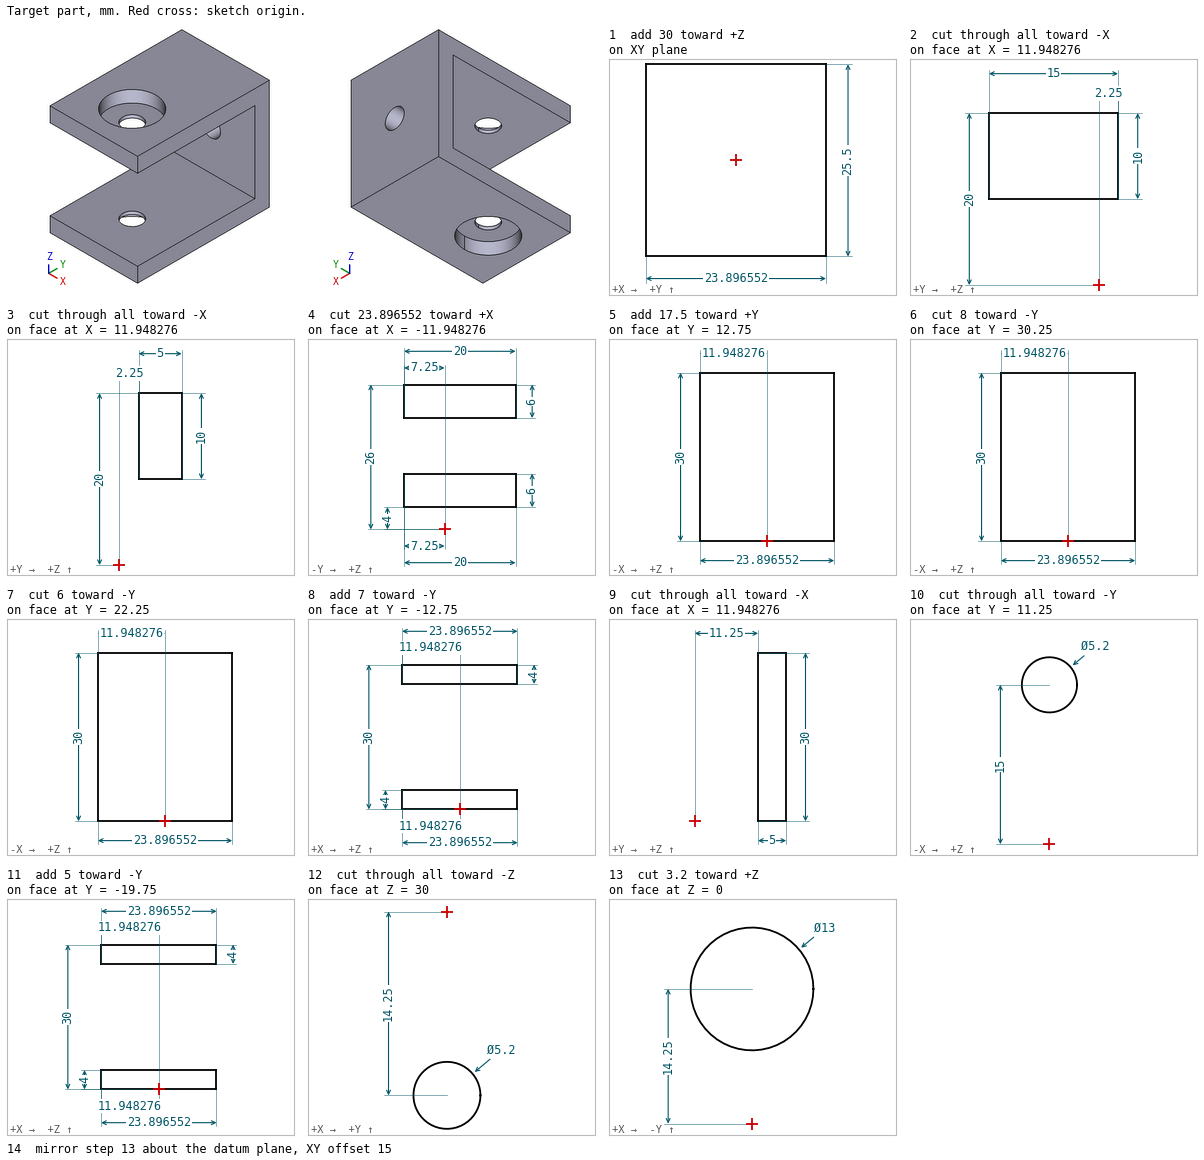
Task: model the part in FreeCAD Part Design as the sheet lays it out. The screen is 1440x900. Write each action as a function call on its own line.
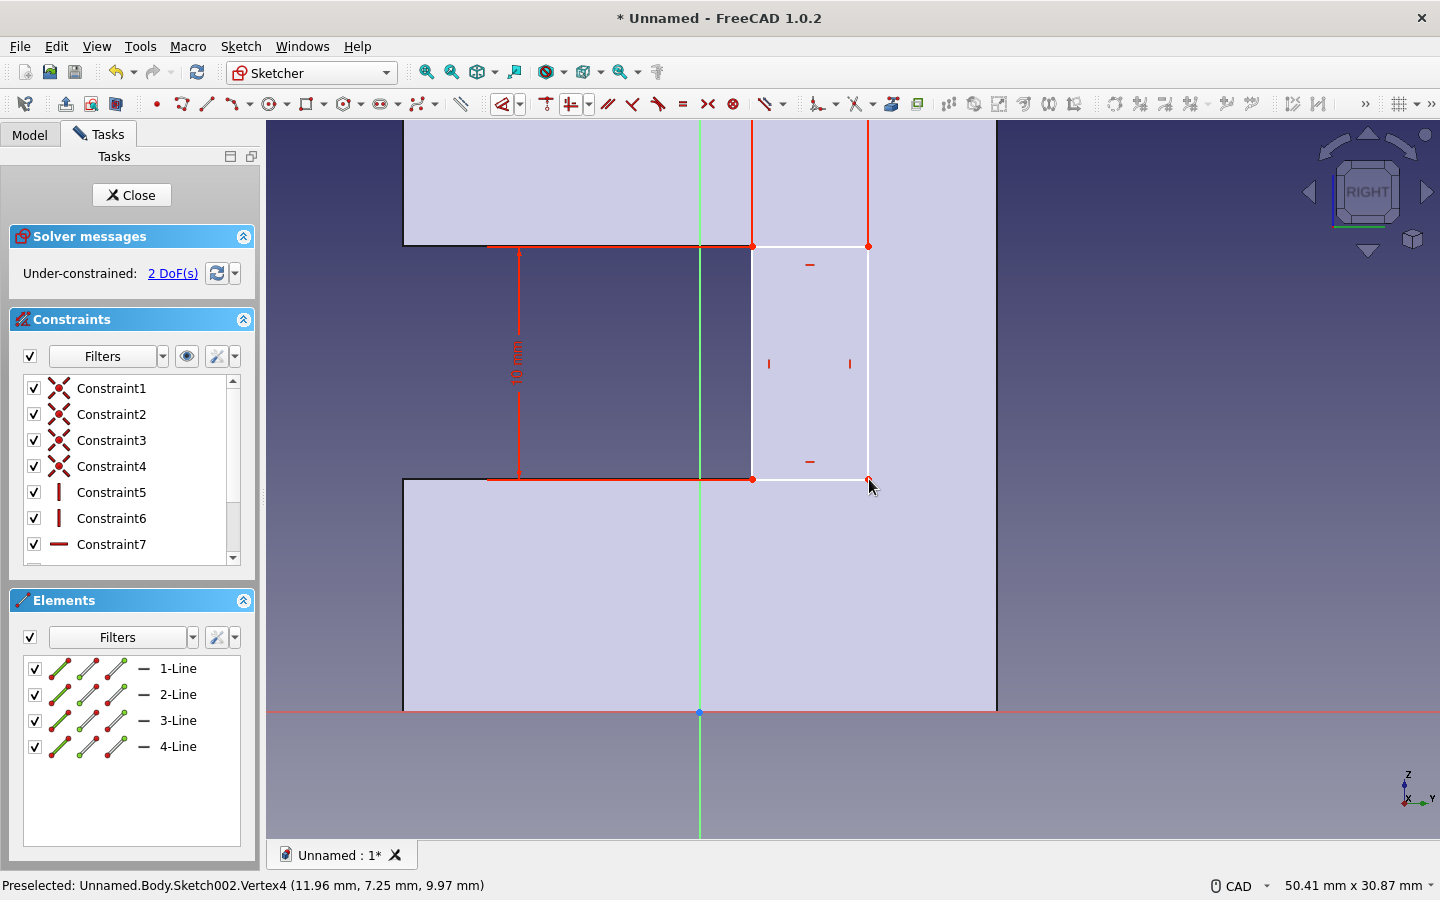
click(502, 104)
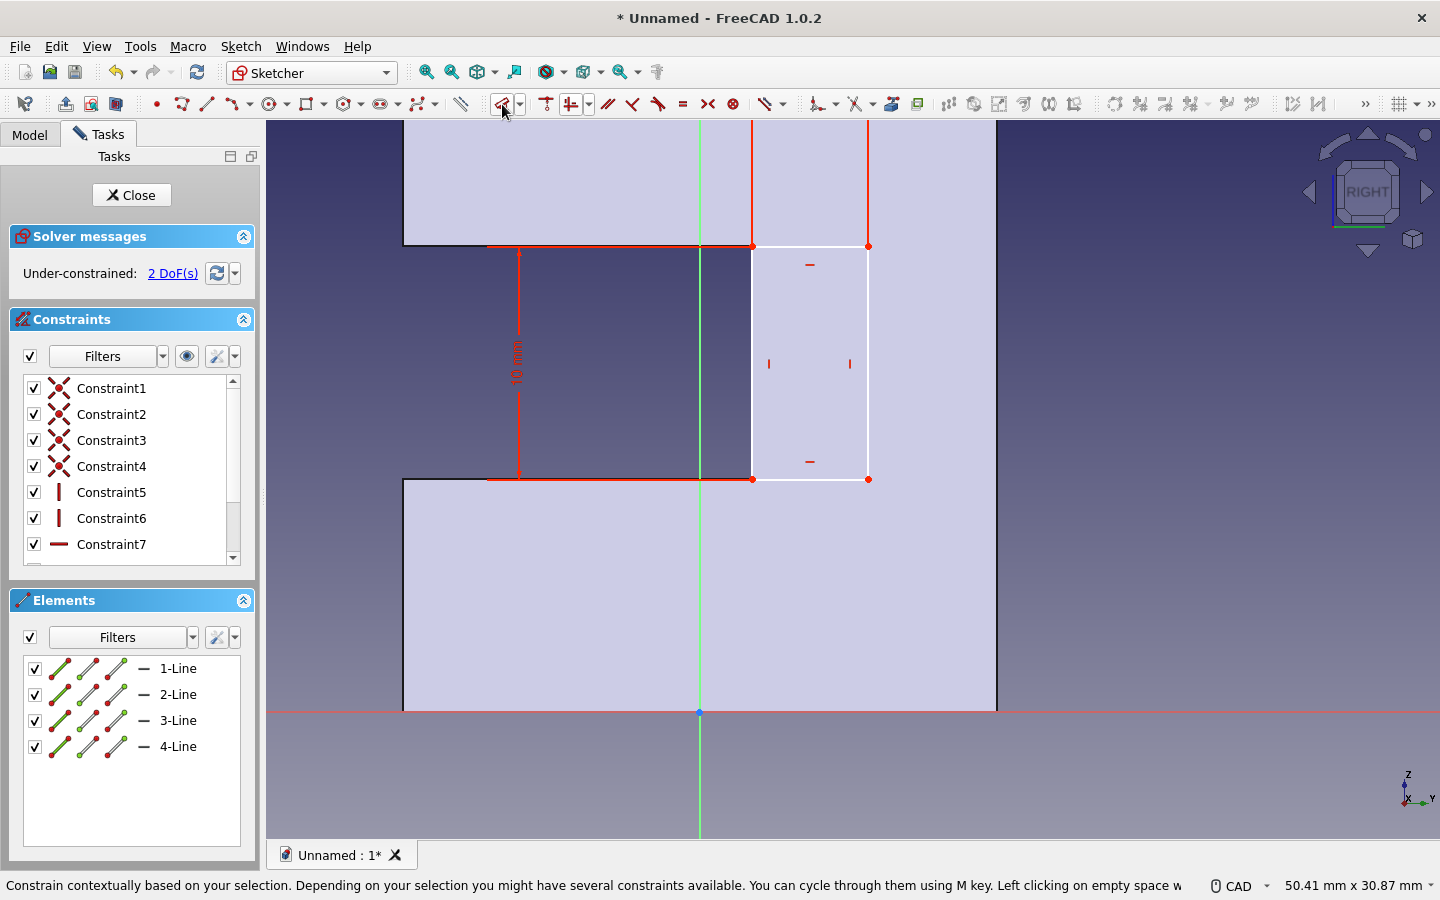
click(752, 247)
click(666, 480)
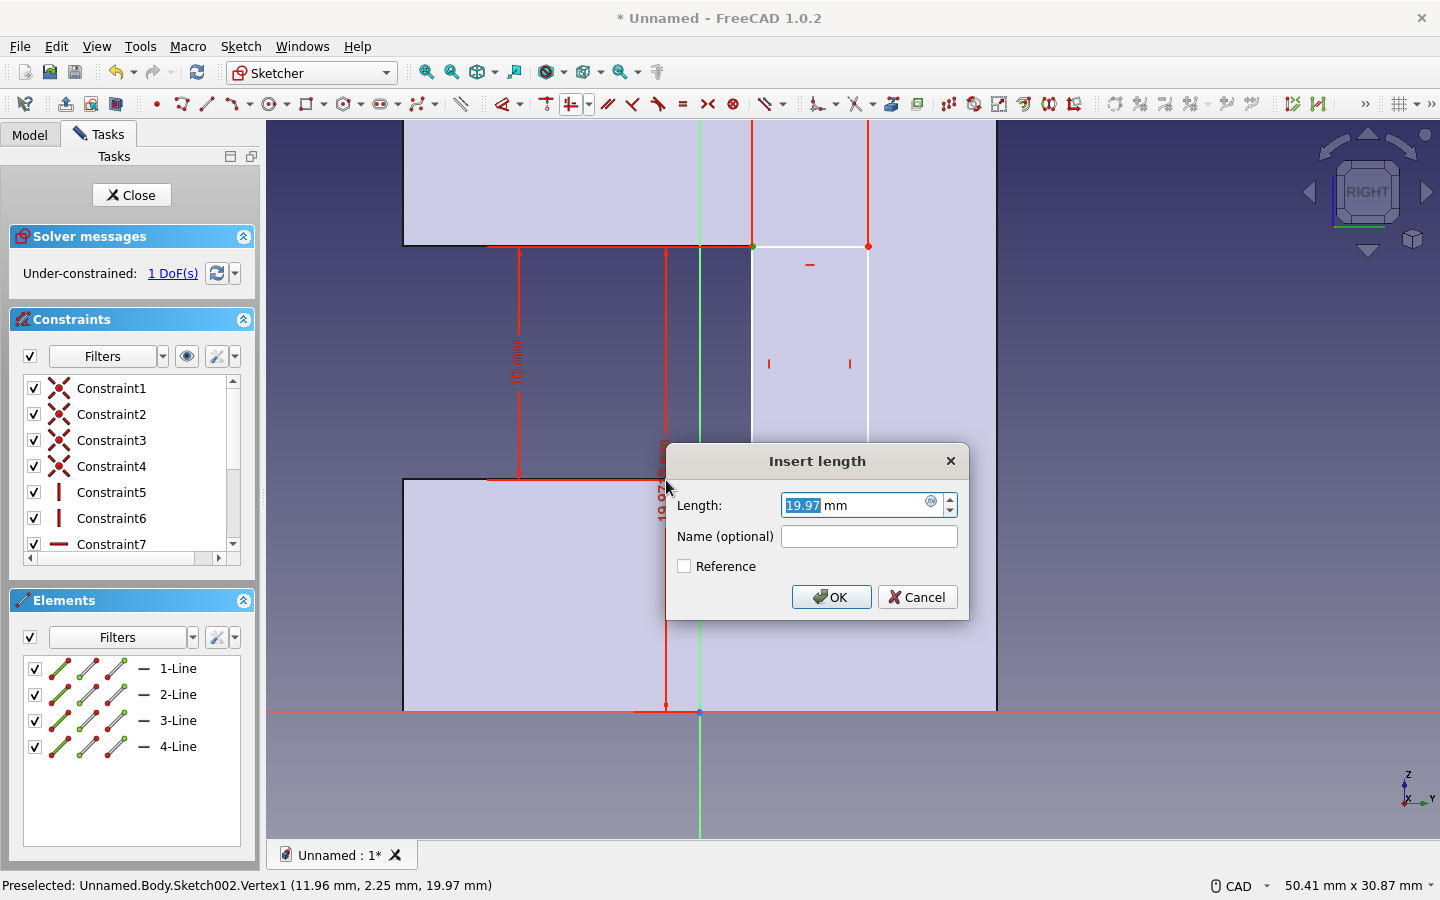
text(20)
key(Return)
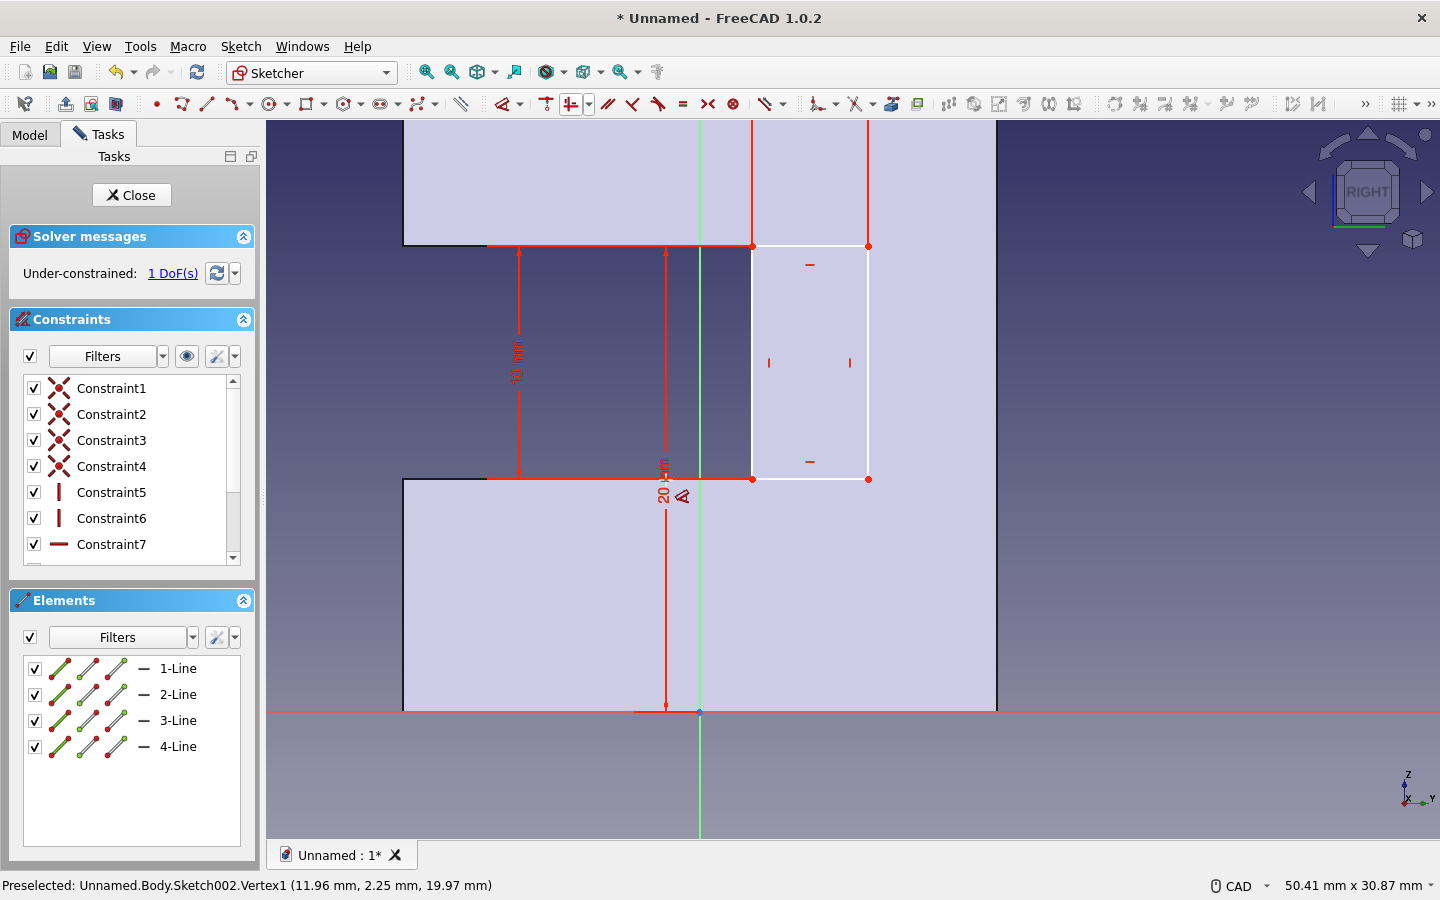
click(752, 246)
click(726, 746)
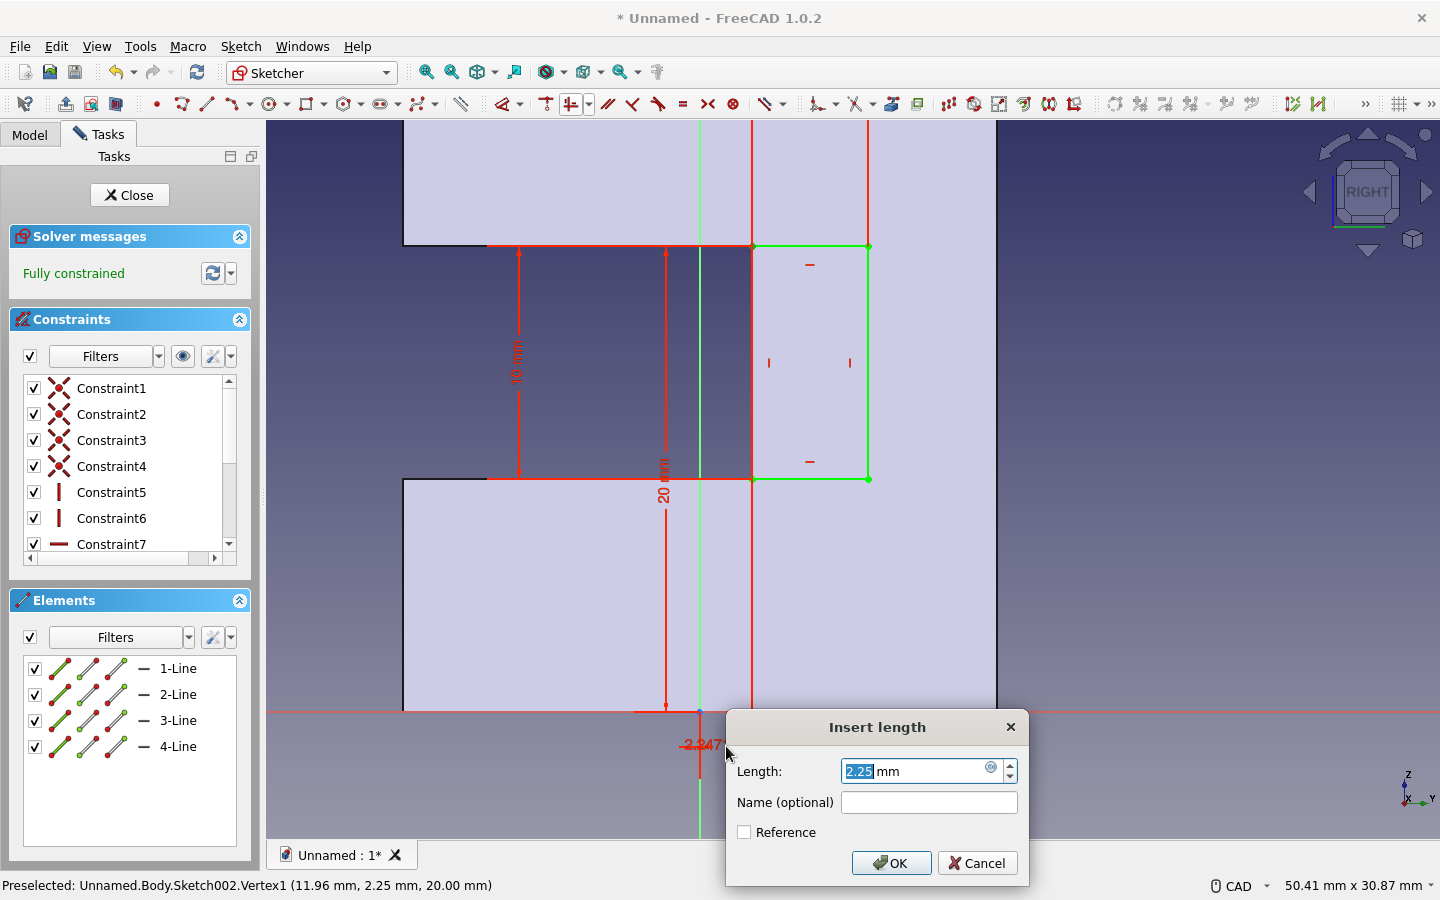
text(2.25)
key(Return)
key(Escape)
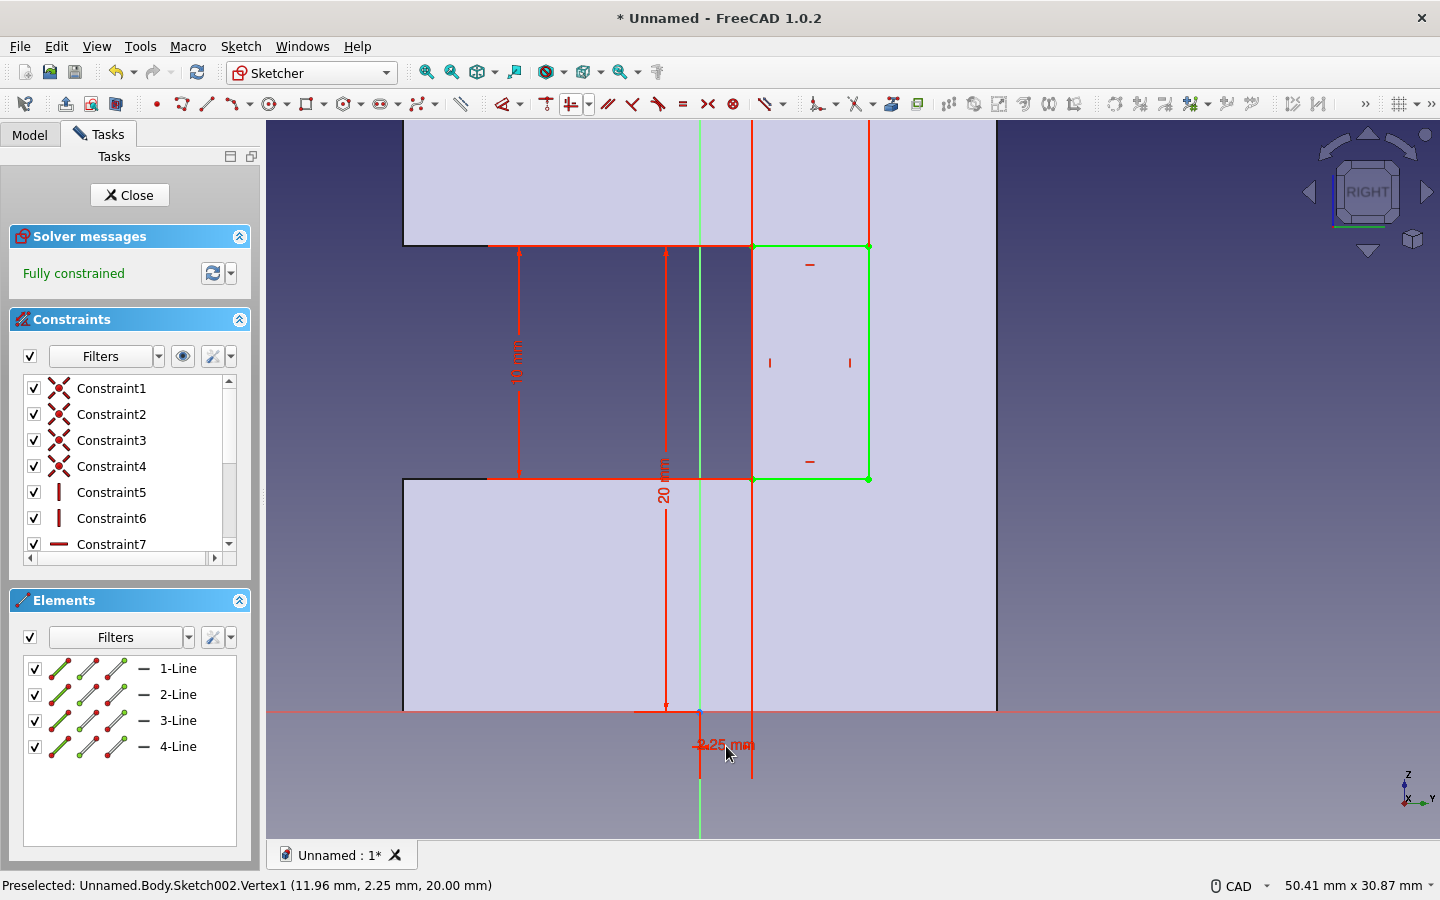
click(130, 195)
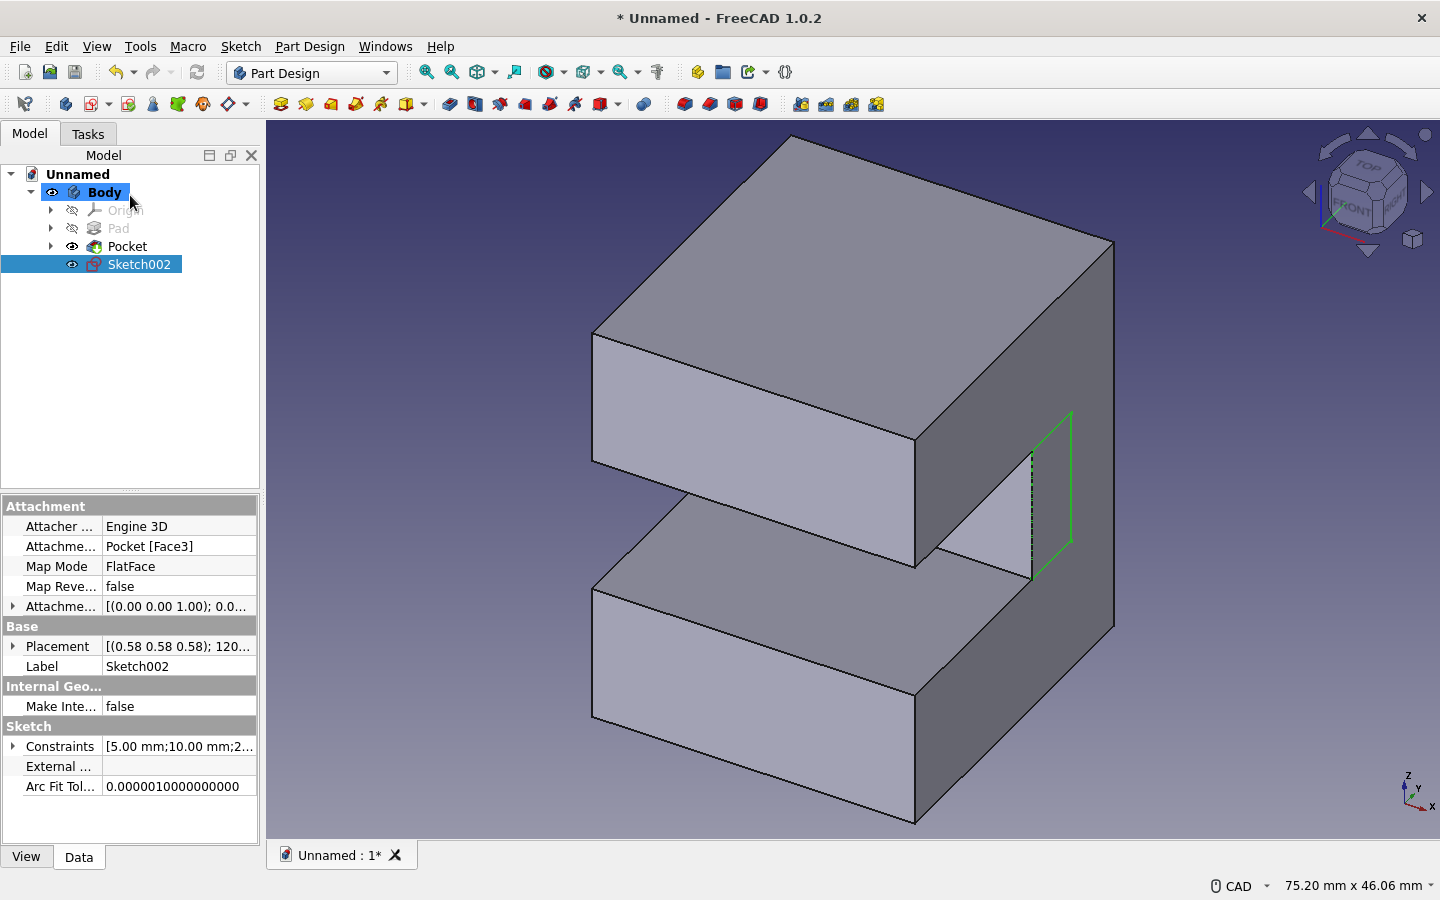
click(450, 104)